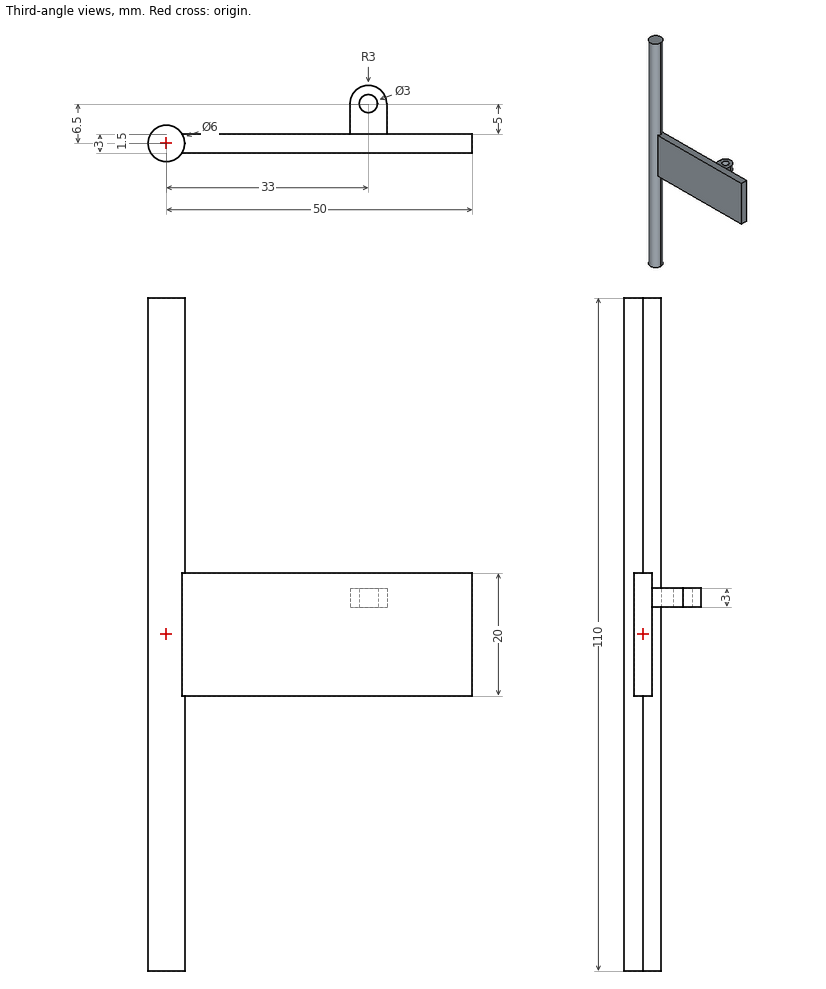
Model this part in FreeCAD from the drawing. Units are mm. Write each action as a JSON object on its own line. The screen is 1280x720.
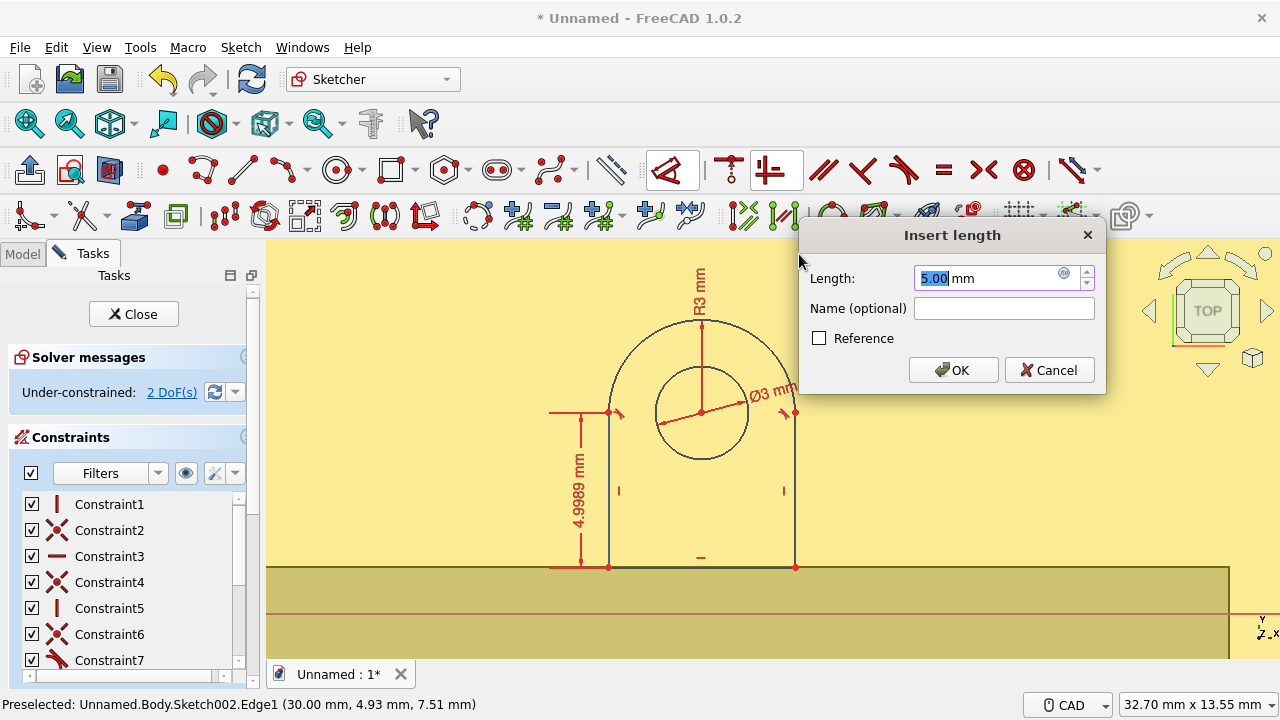
{"action": "type", "text": "5"}
{"action": "key", "text": "Return"}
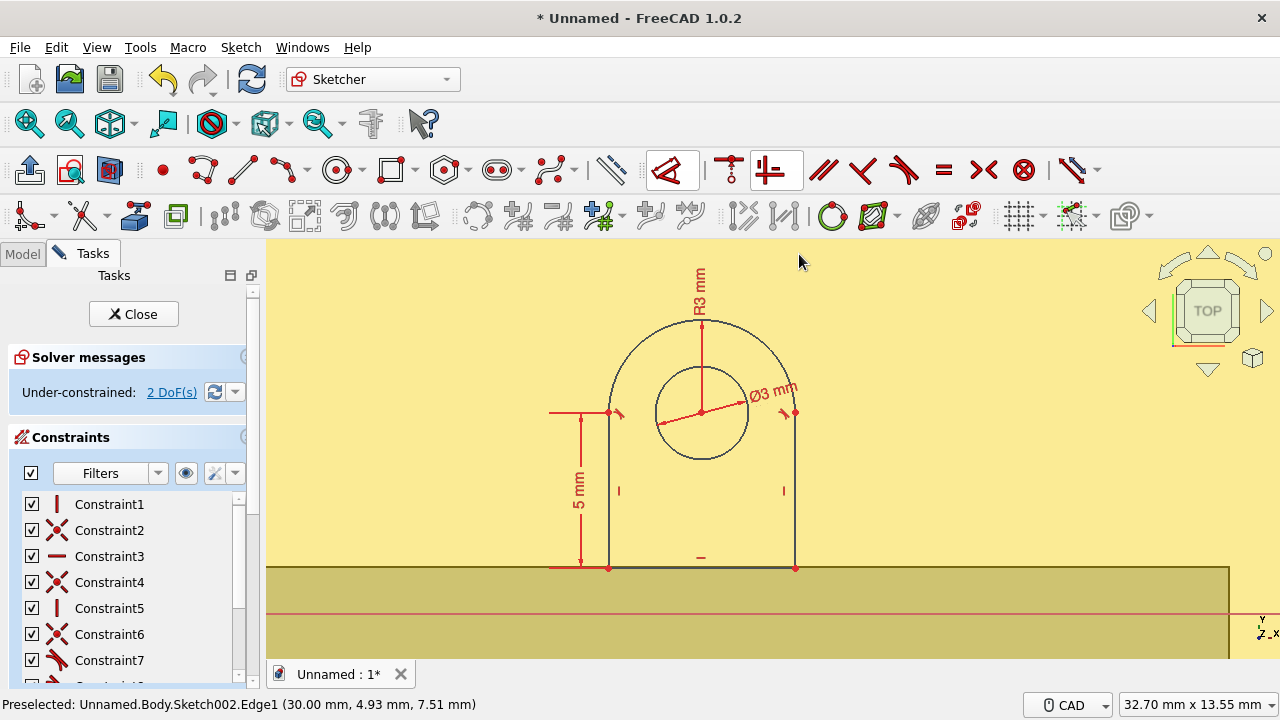
{"action": "left_click", "coordinate": [702, 413]}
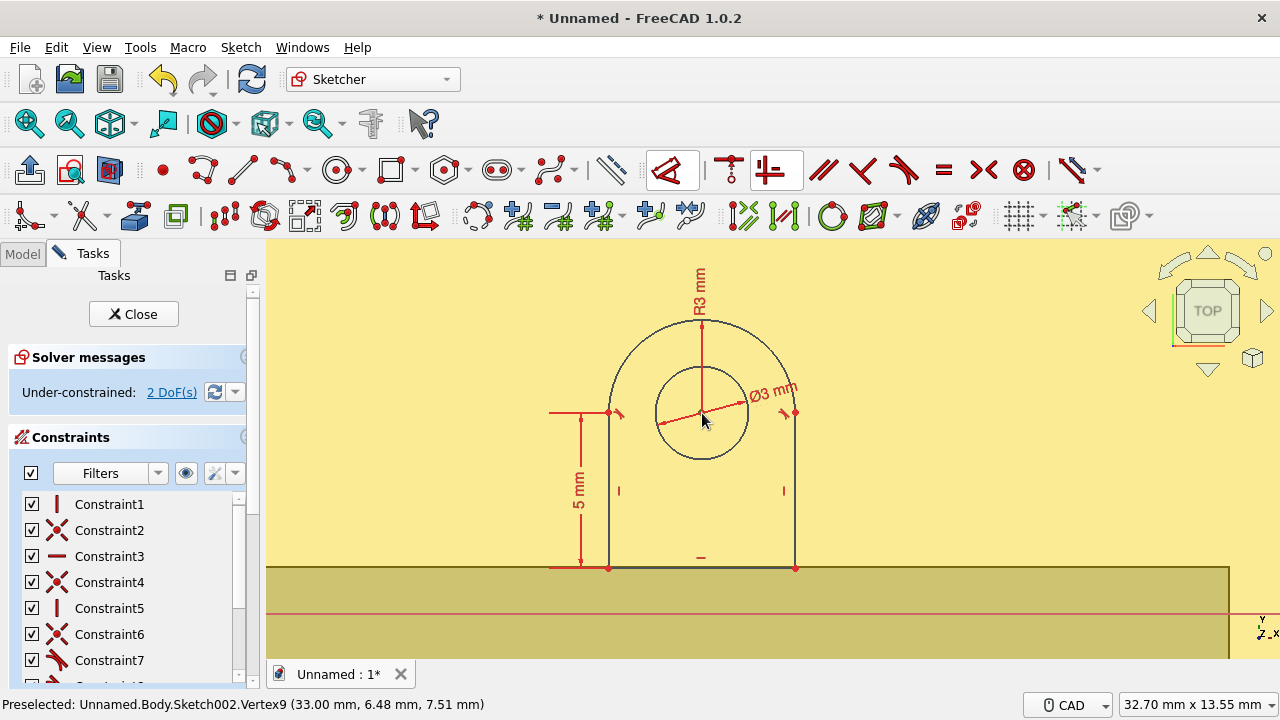
{"action": "key", "text": "l"}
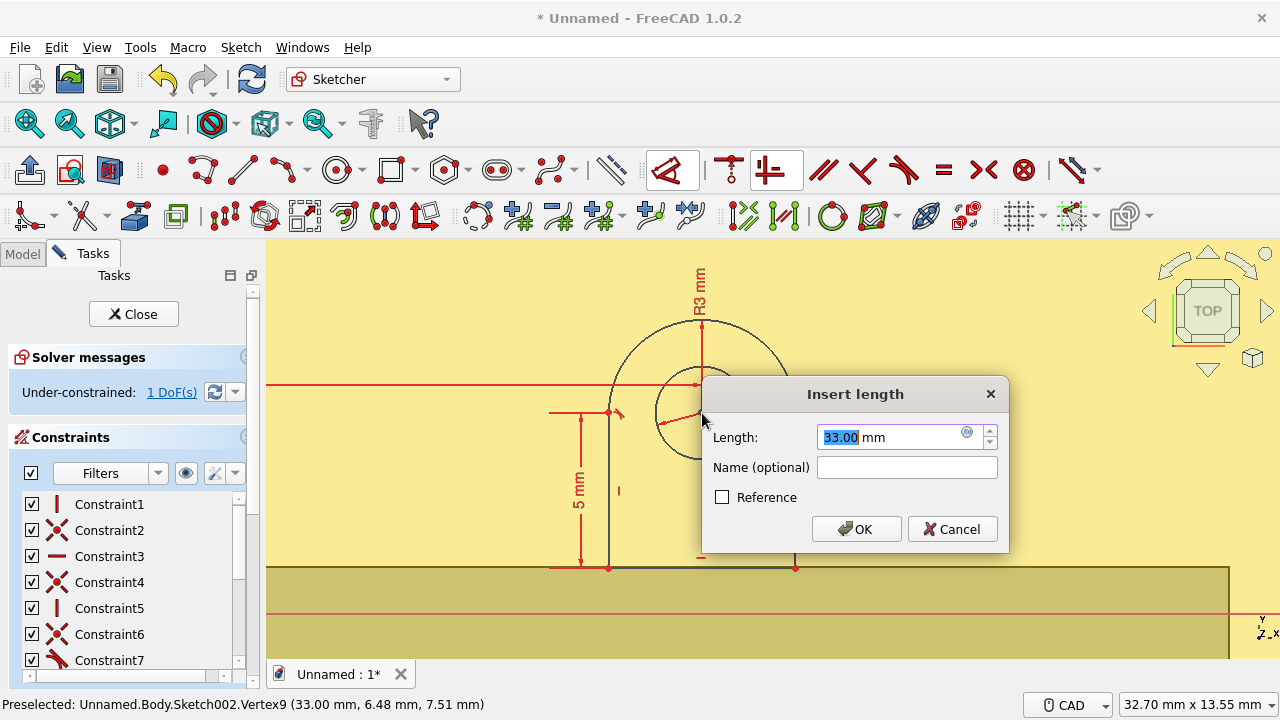
{"action": "type", "text": "33"}
{"action": "key", "text": "Return"}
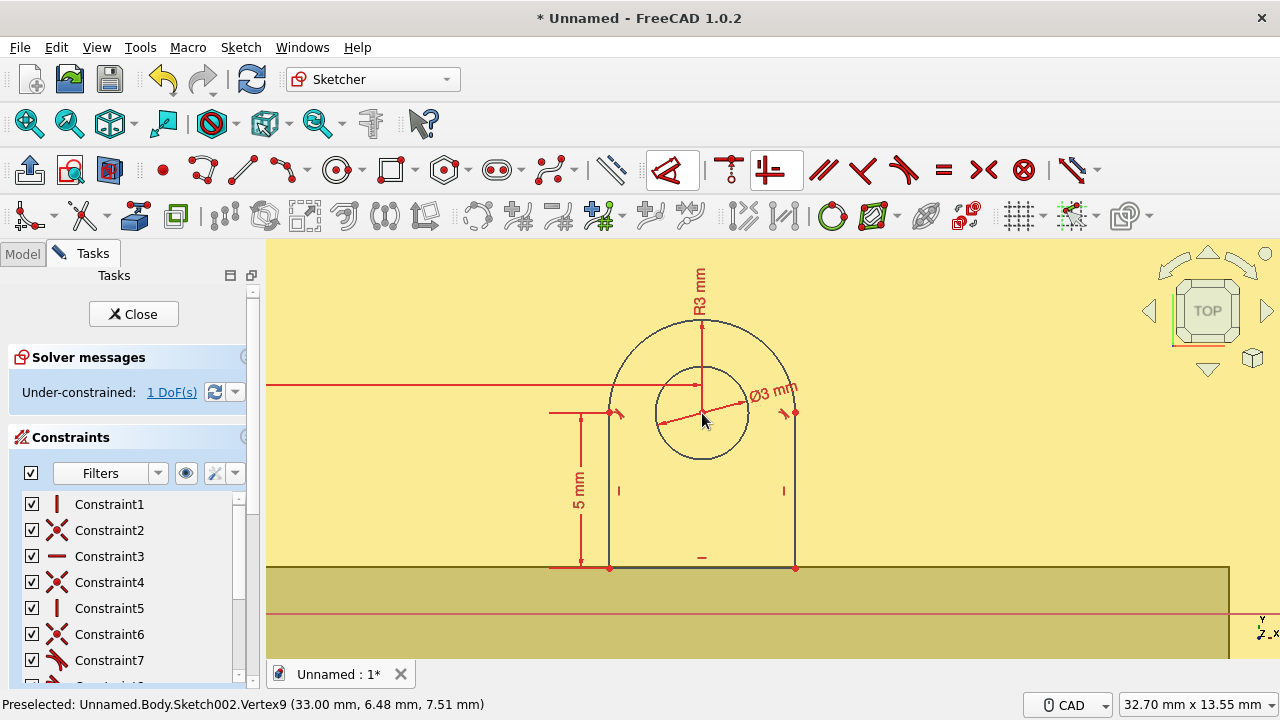
{"action": "left_click", "coordinate": [702, 413]}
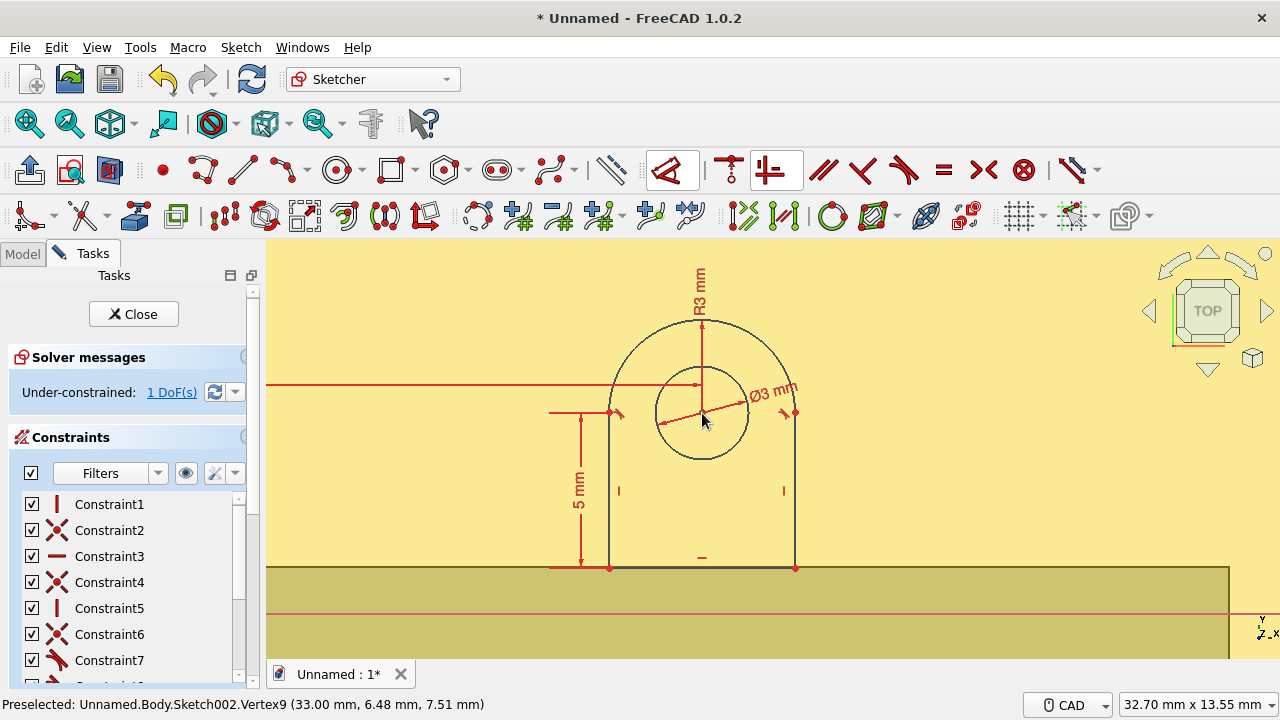
{"action": "key", "text": "i"}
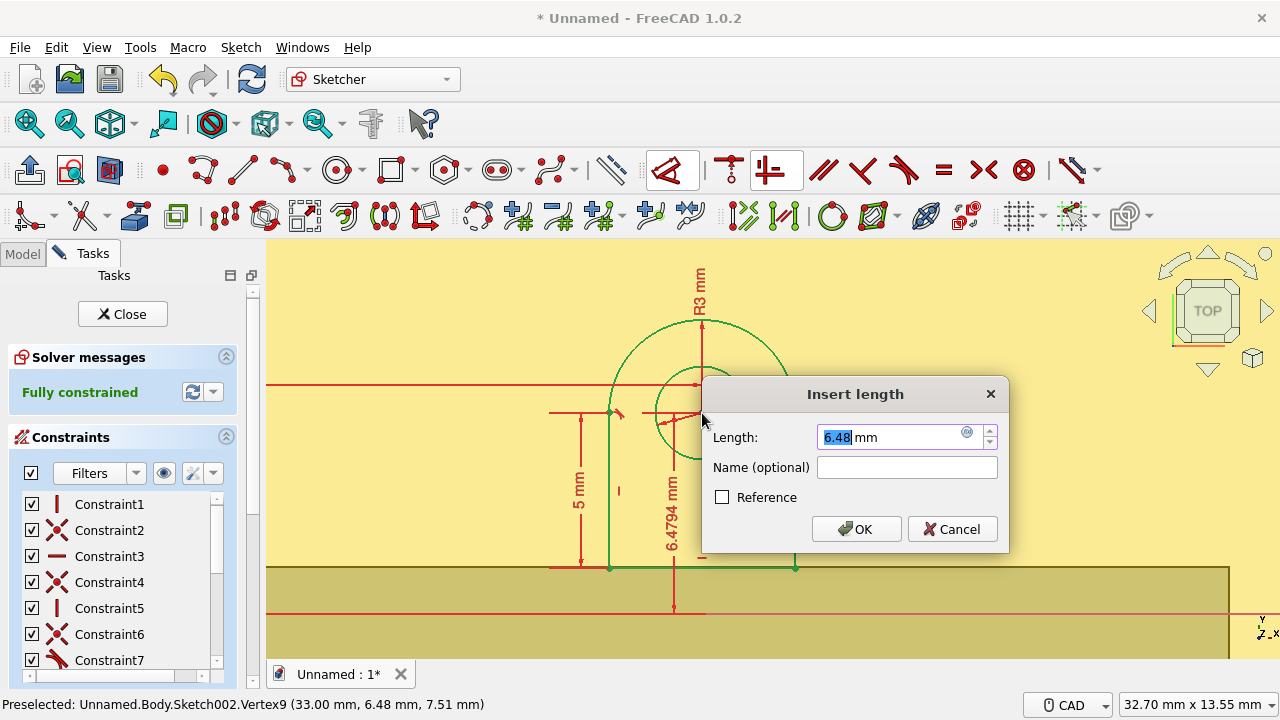
{"action": "type", "text": "6.5"}
{"action": "key", "text": "Return"}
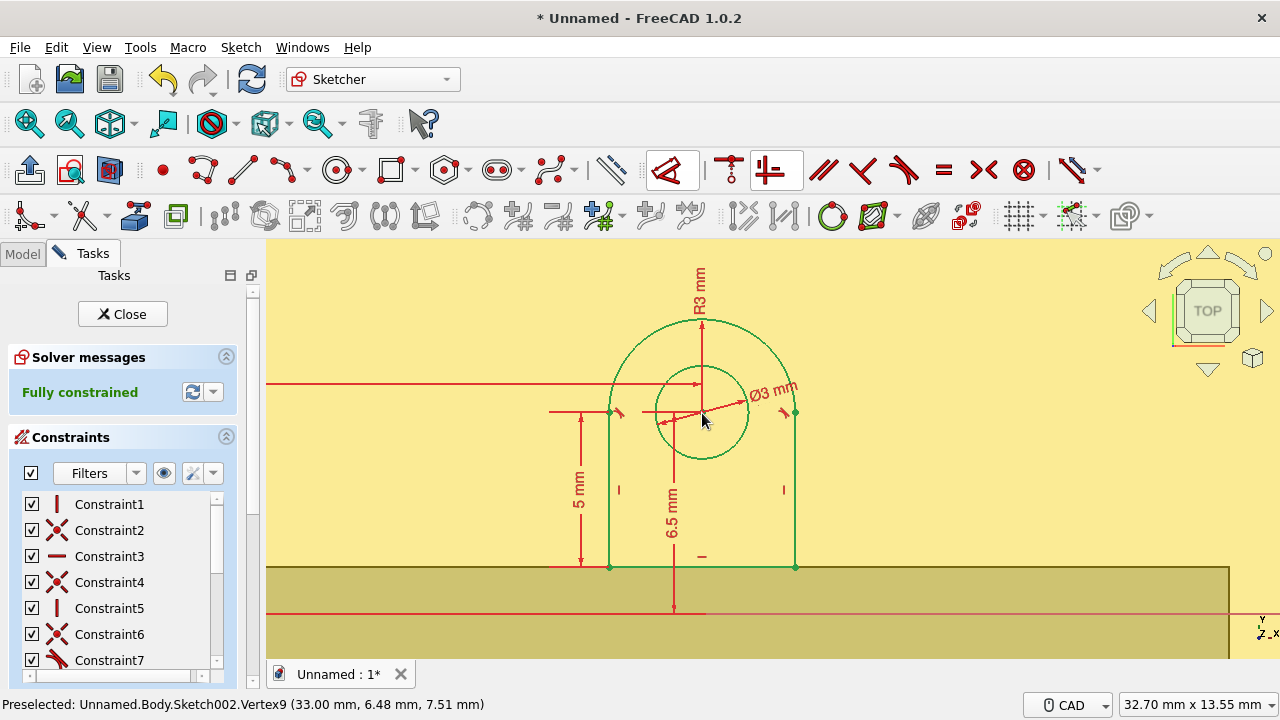
{"action": "left_click", "coordinate": [123, 314]}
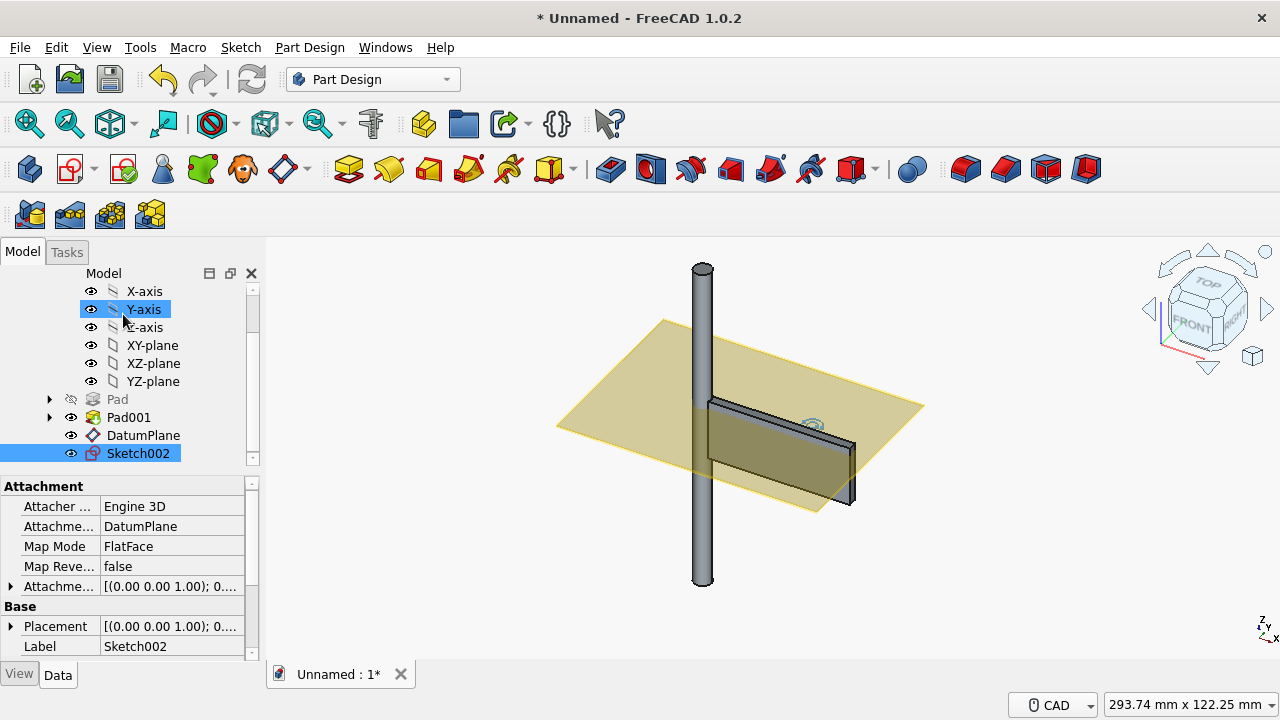
{"action": "left_click", "coordinate": [350, 170]}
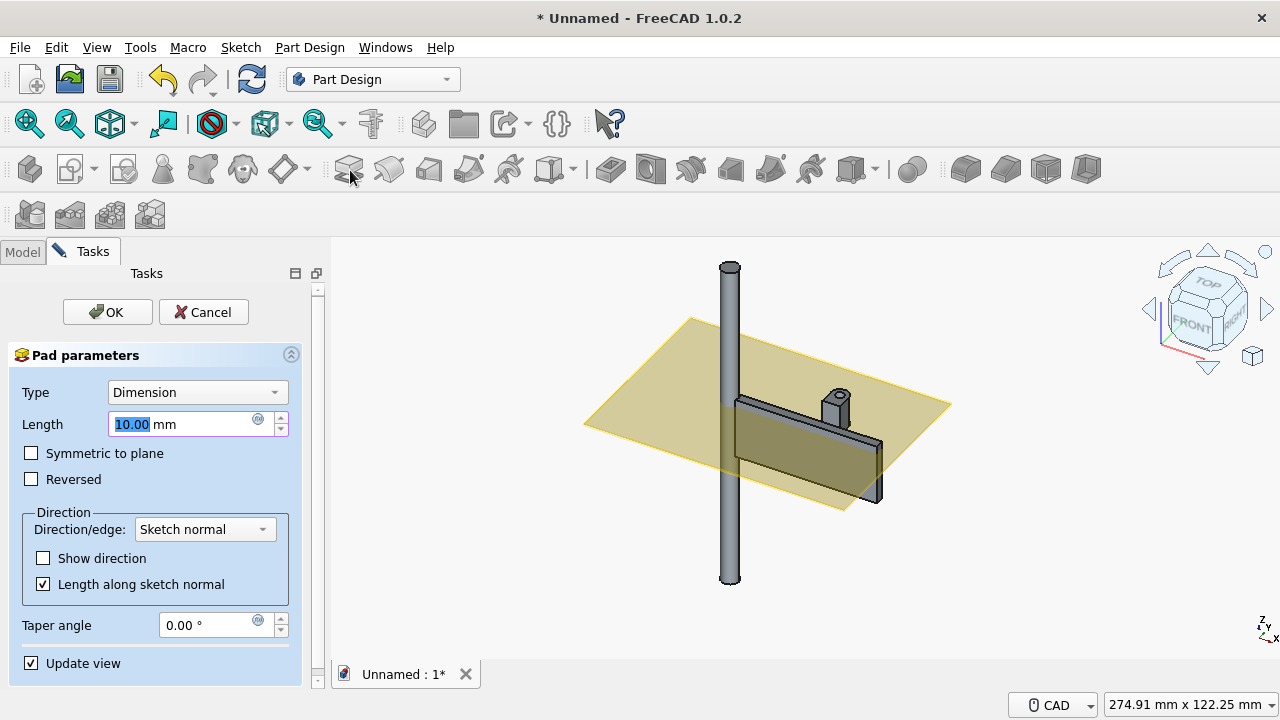
{"action": "type", "text": "3"}
{"action": "key", "text": "Tab"}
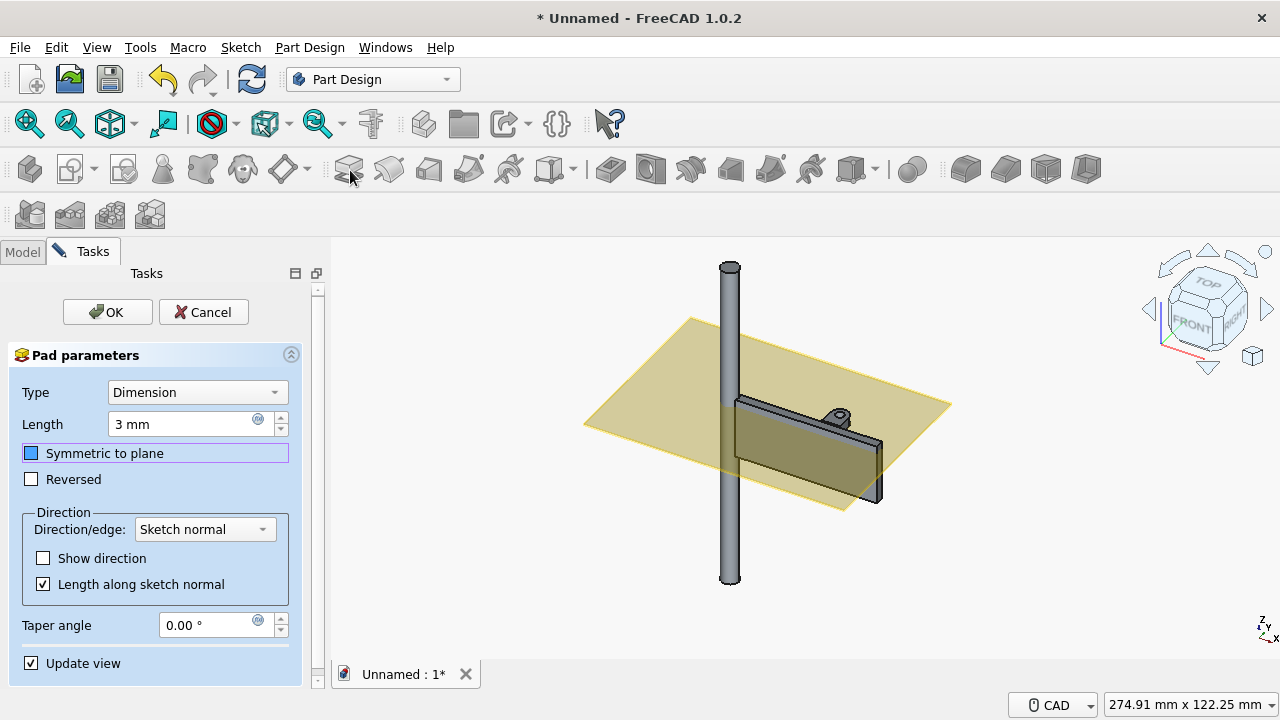
{"action": "left_click", "coordinate": [30, 479]}